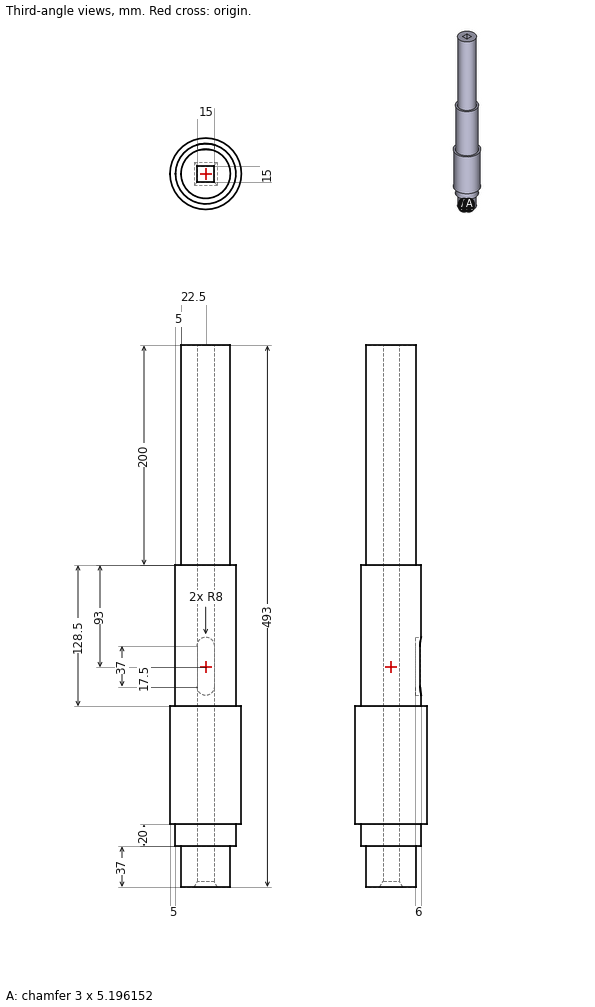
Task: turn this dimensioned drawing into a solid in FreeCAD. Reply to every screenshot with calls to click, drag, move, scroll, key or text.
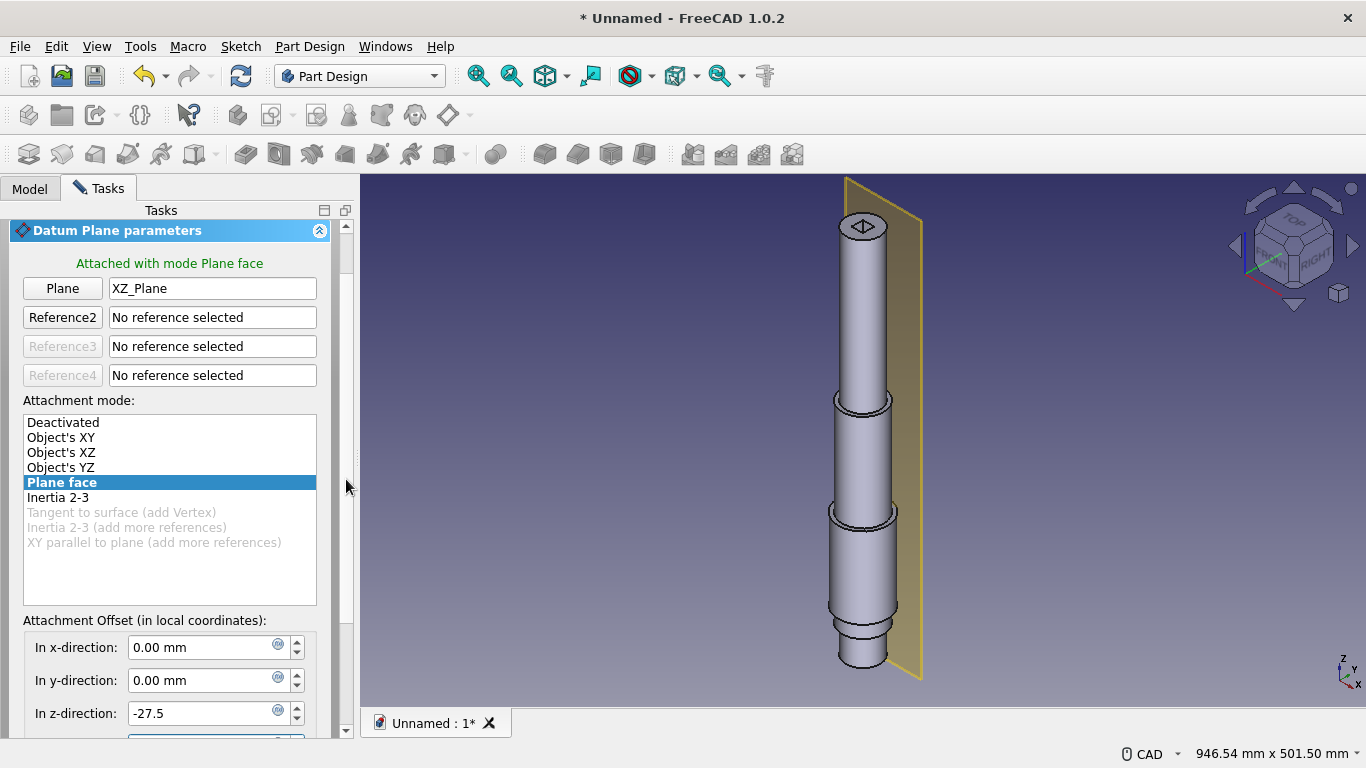
click(127, 249)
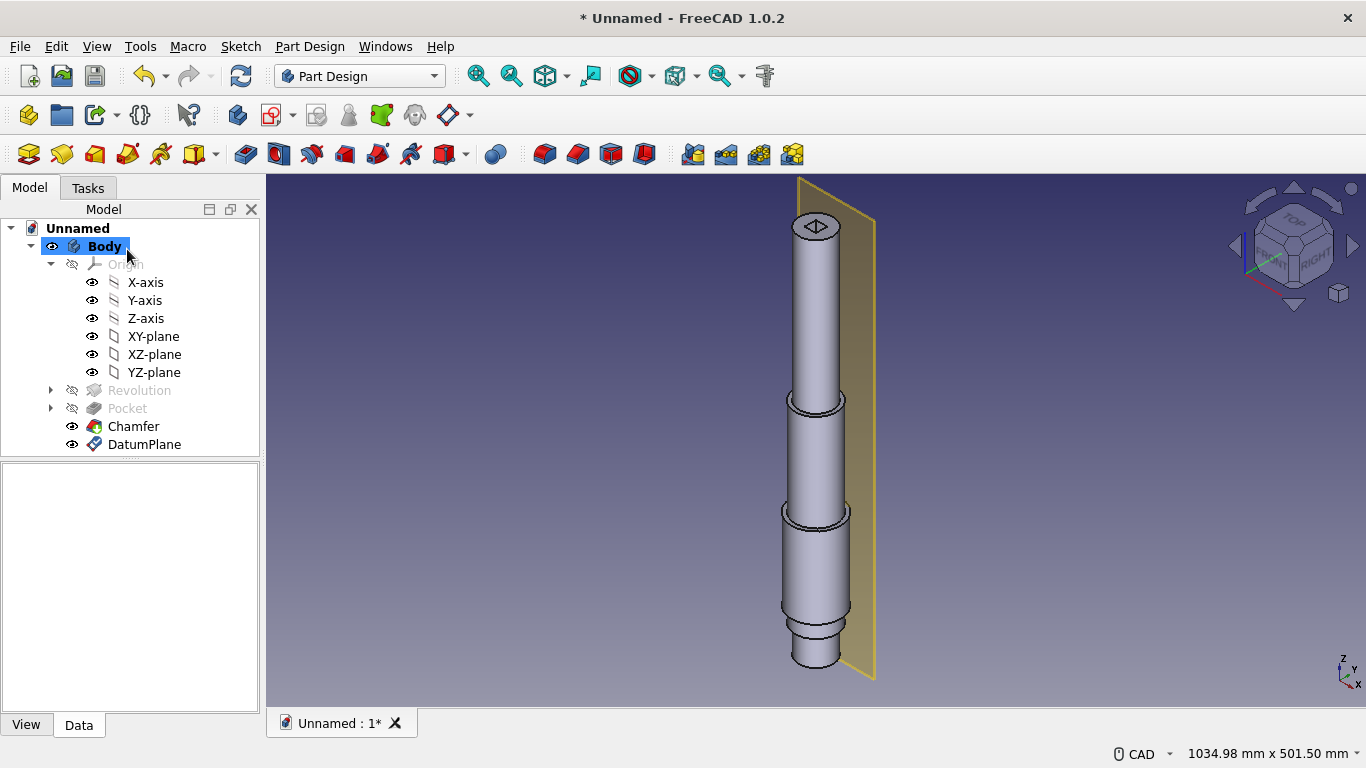
click(117, 444)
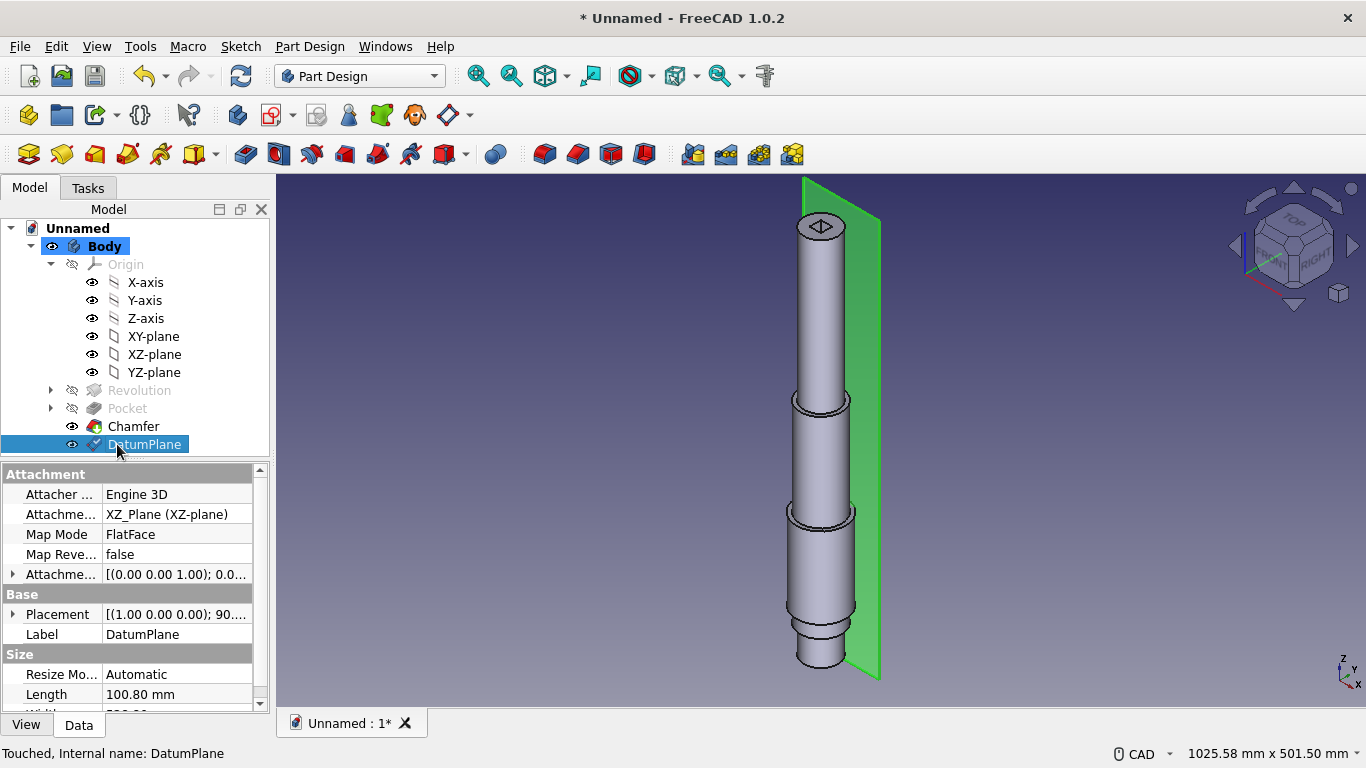
click(270, 116)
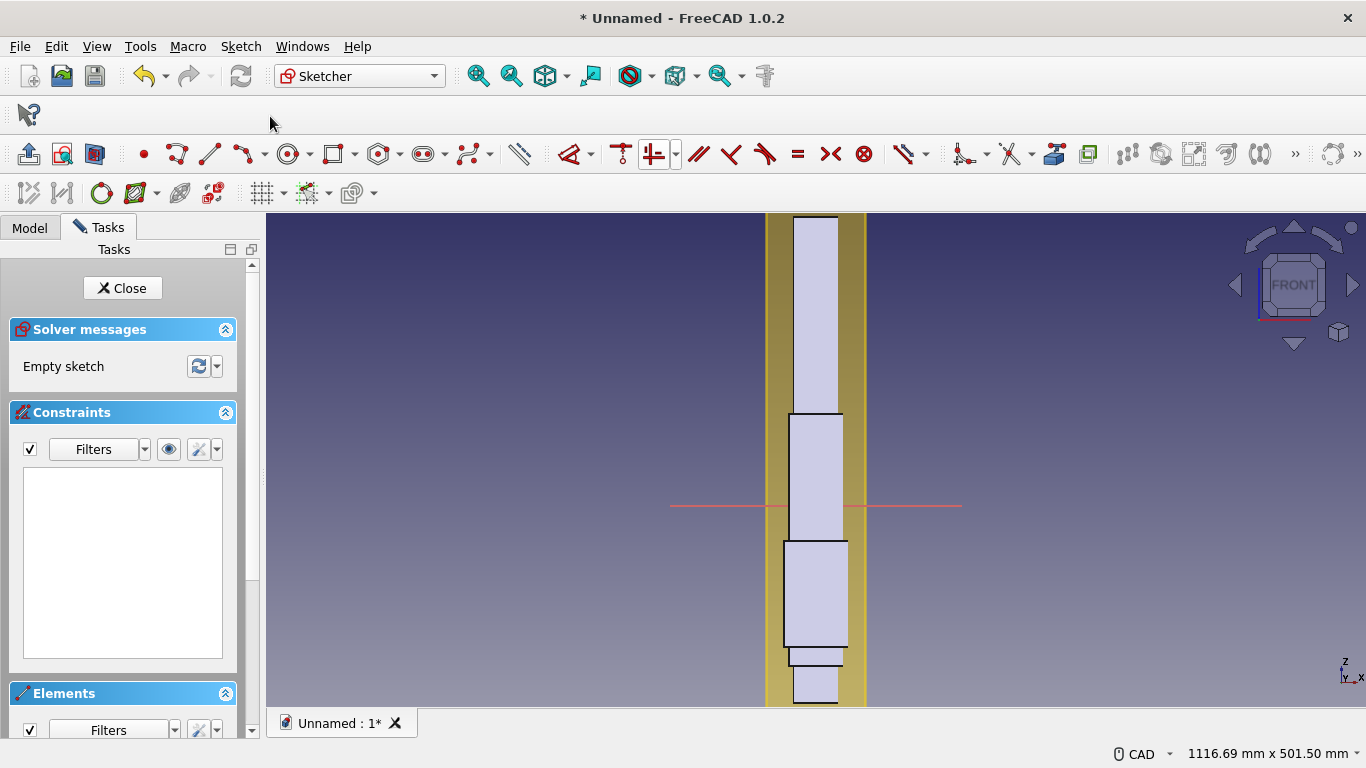
click(95, 154)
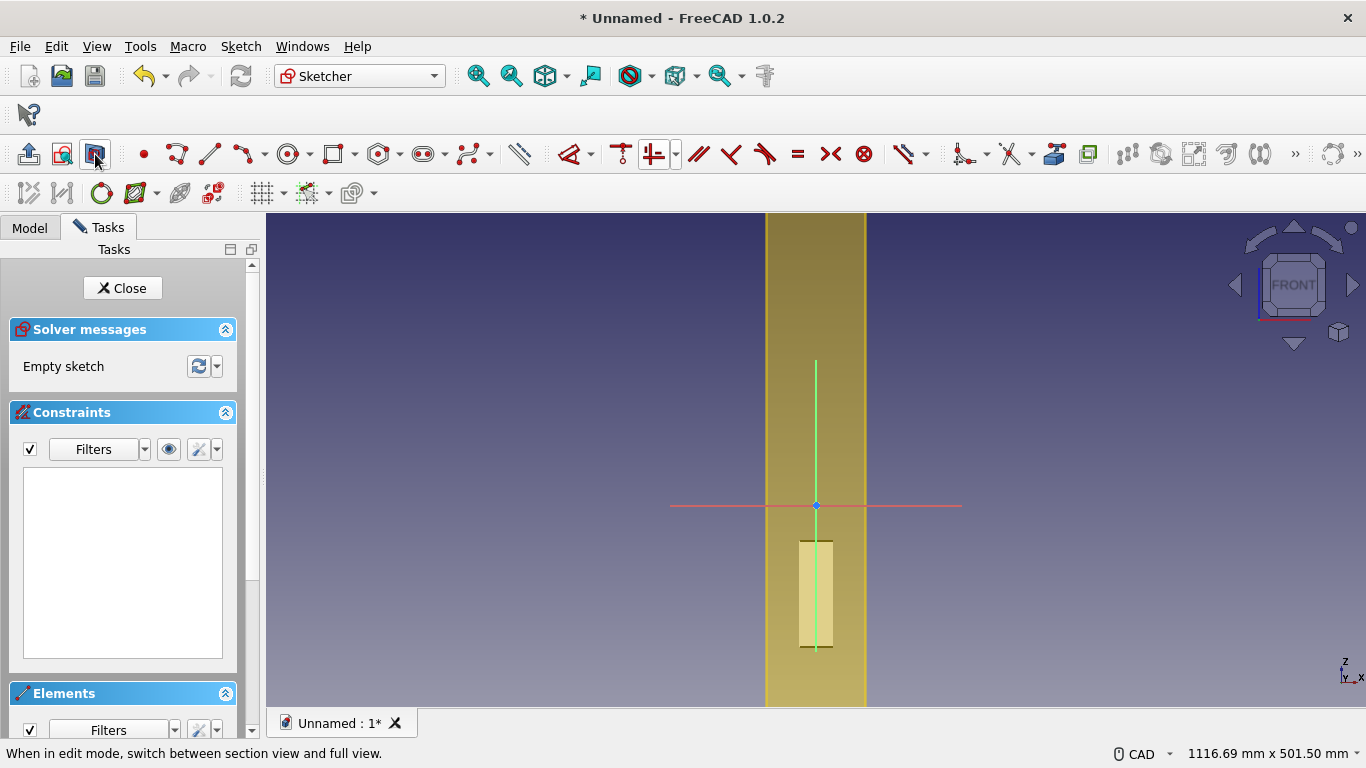
scroll(830, 514, up, 9)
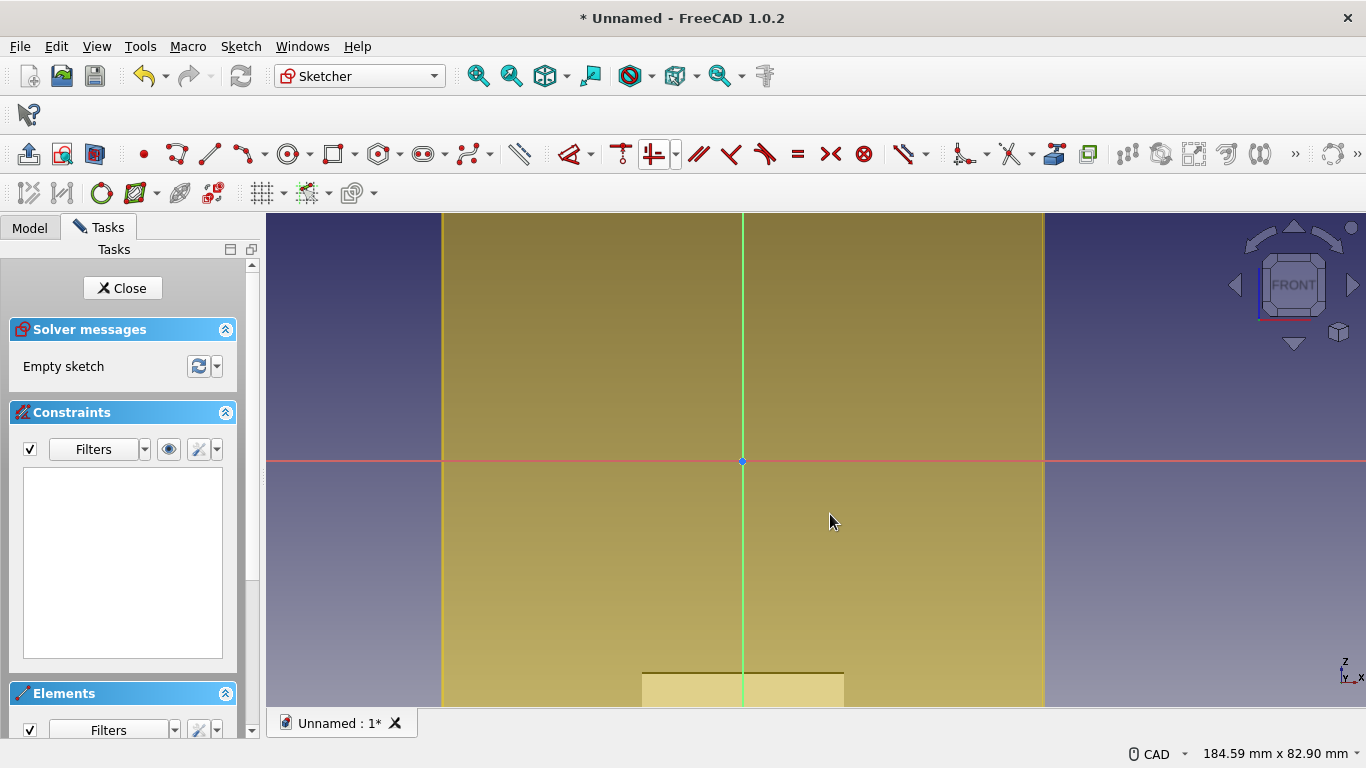
click(422, 154)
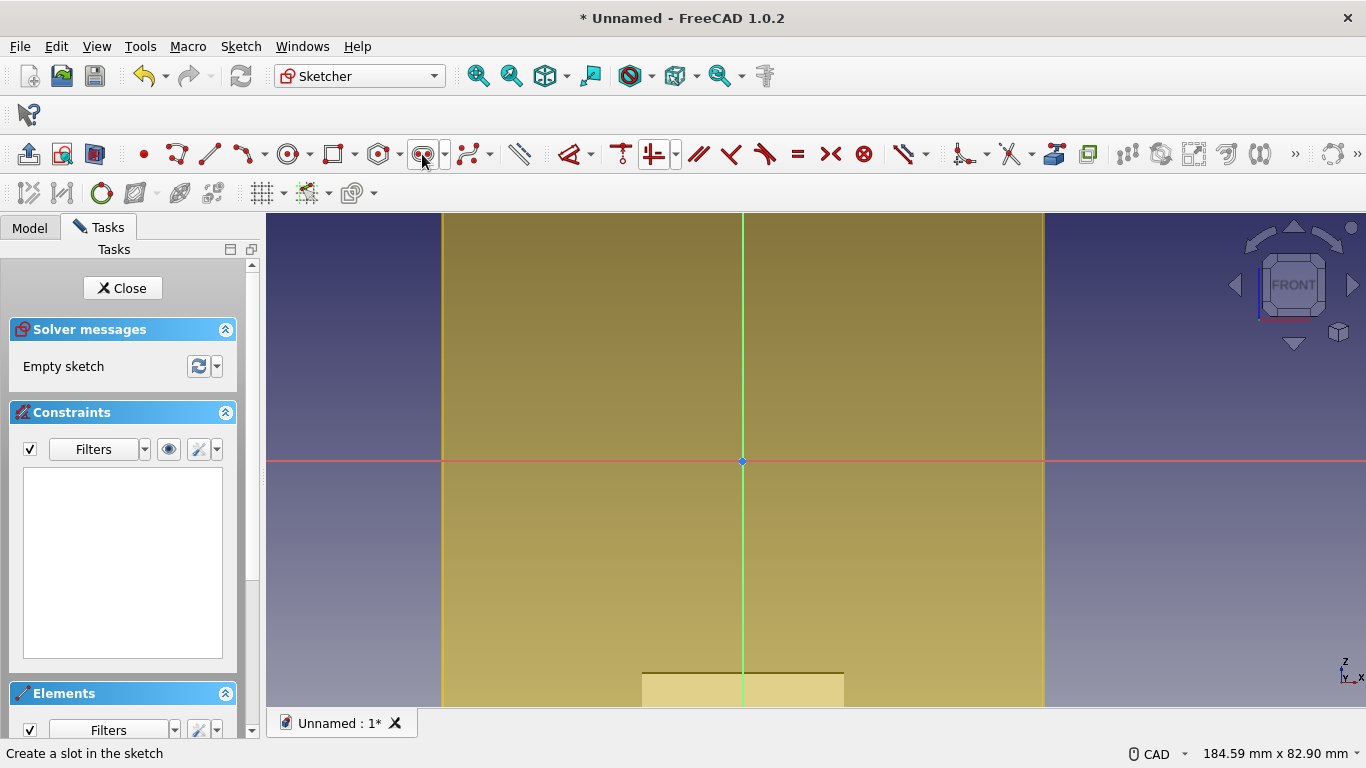
click(743, 566)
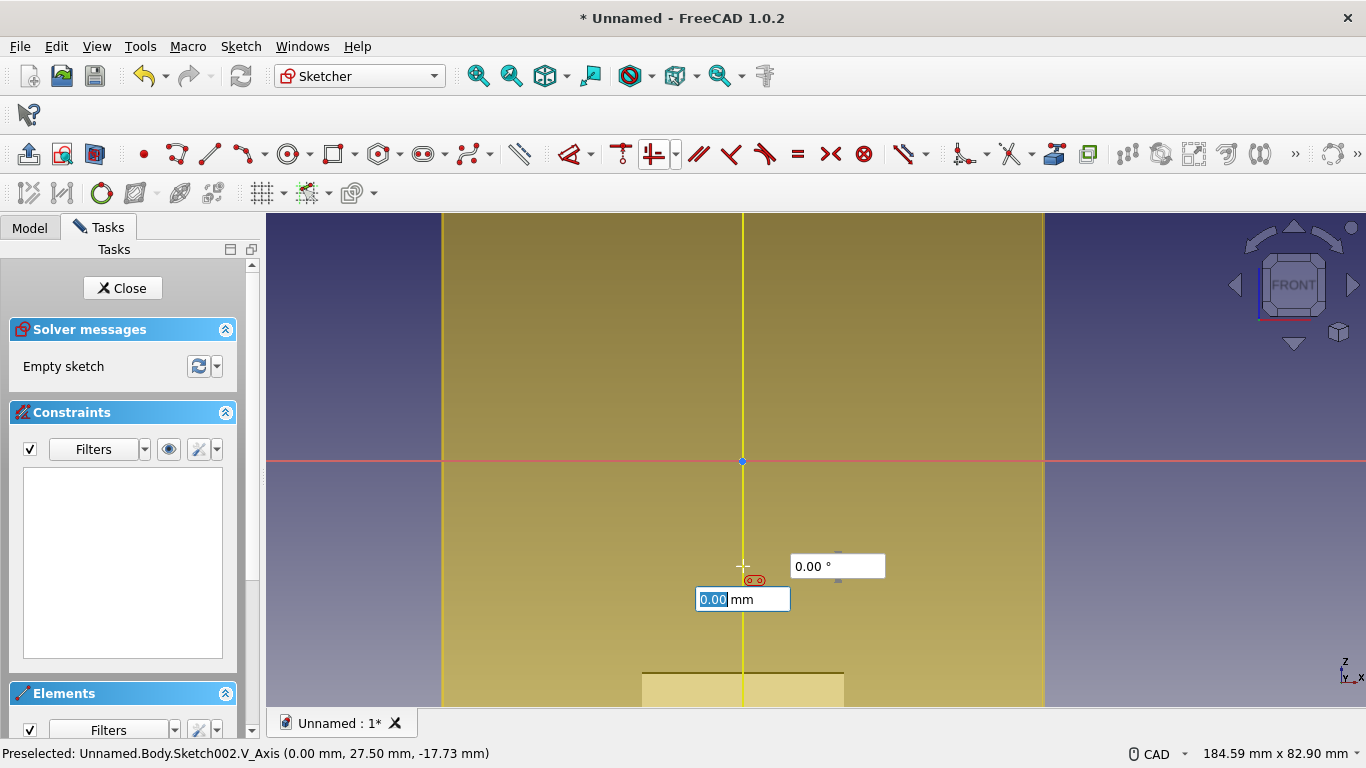
click(752, 345)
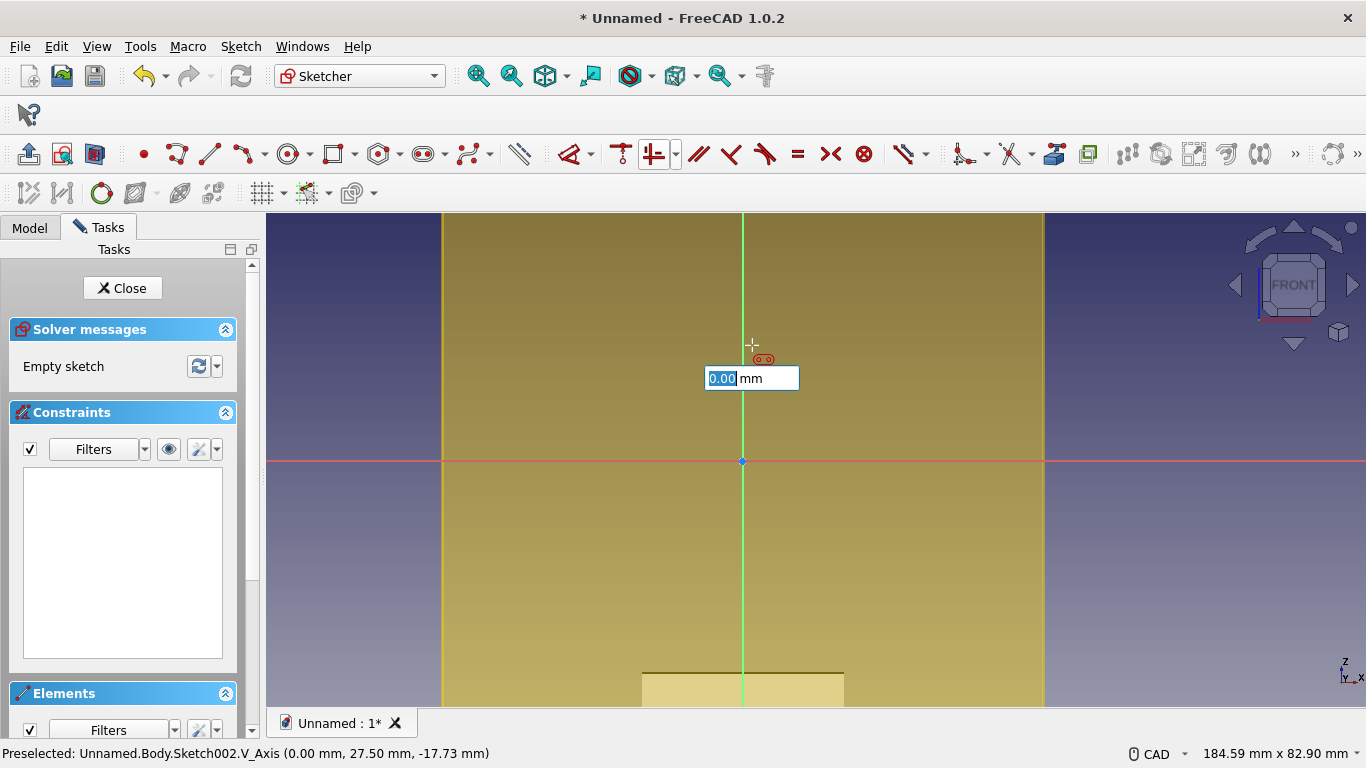
click(695, 488)
key(Escape)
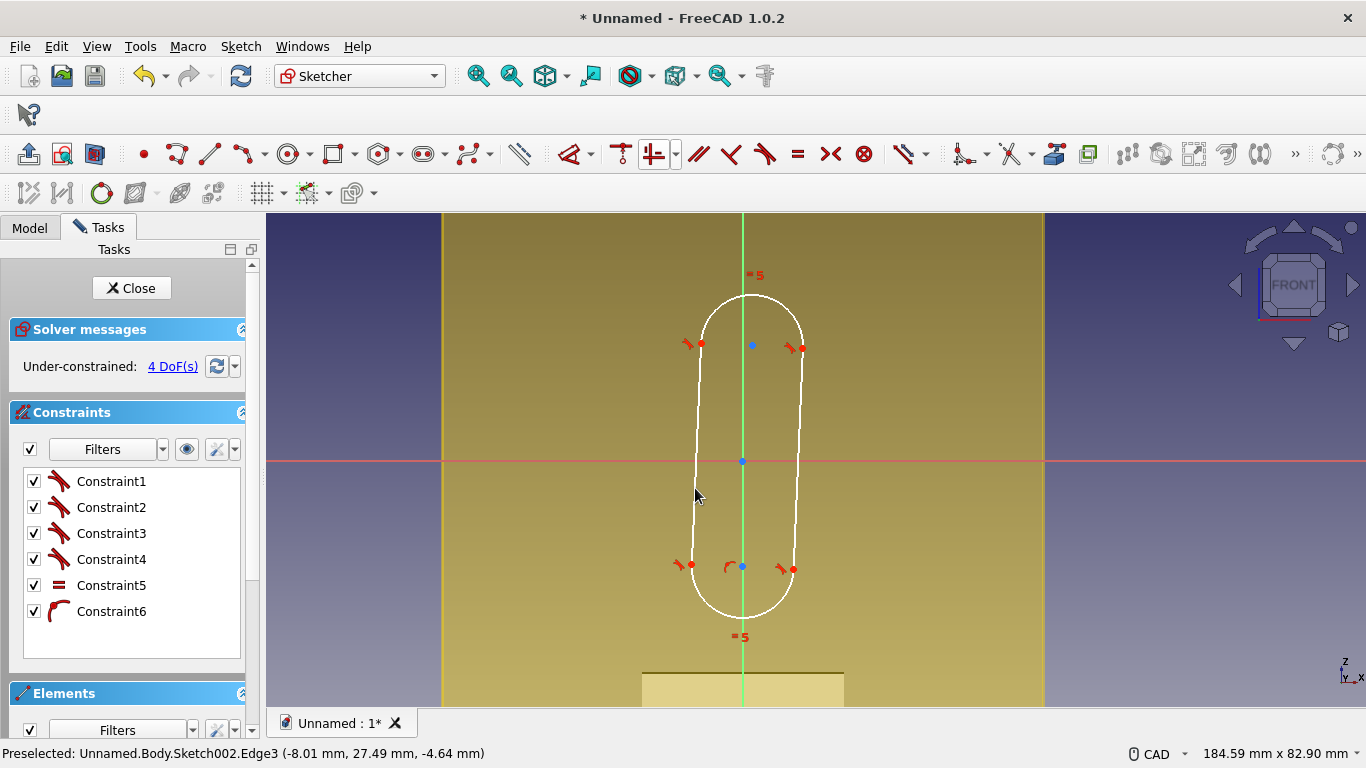
click(695, 499)